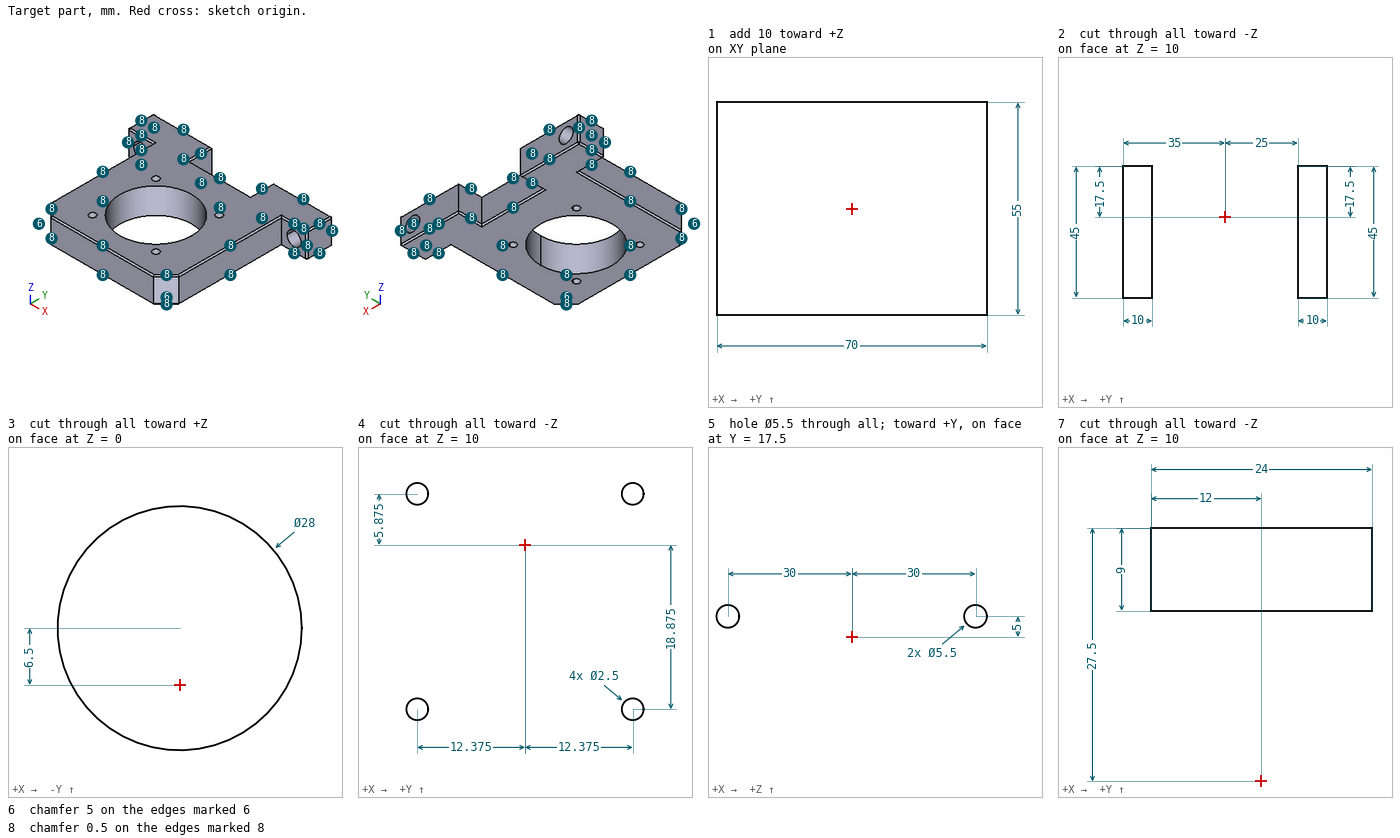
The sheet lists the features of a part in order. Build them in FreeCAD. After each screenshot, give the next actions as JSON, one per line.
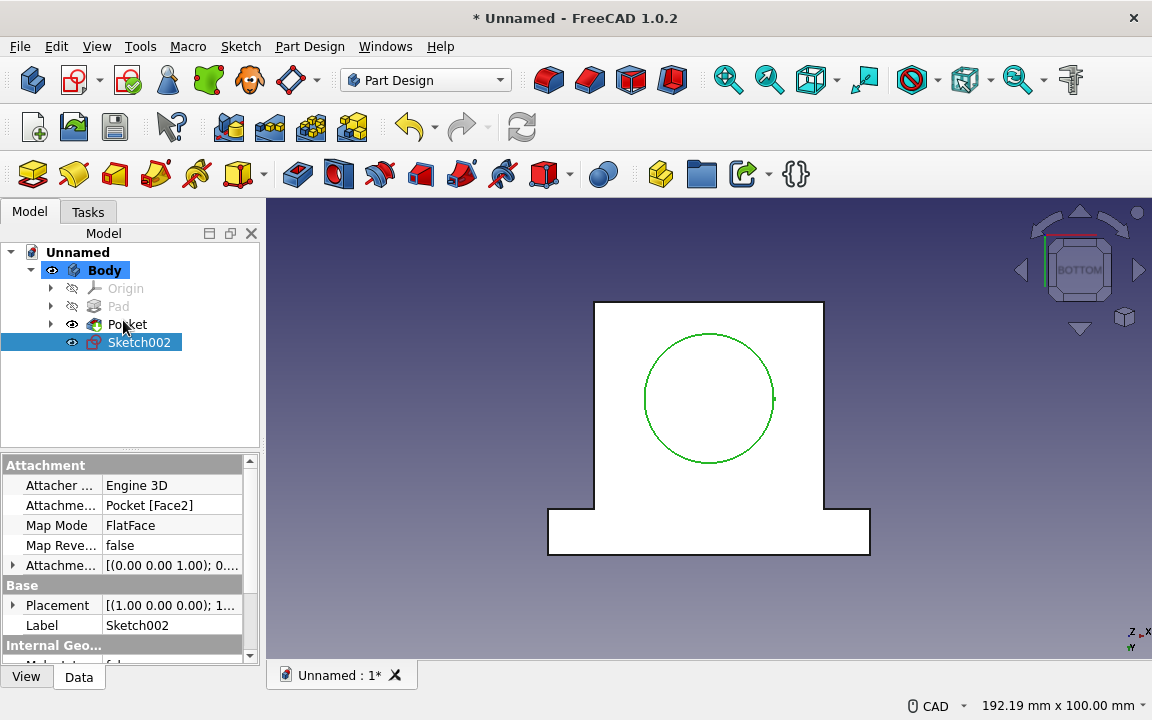
{"action": "left_click", "coordinate": [298, 174]}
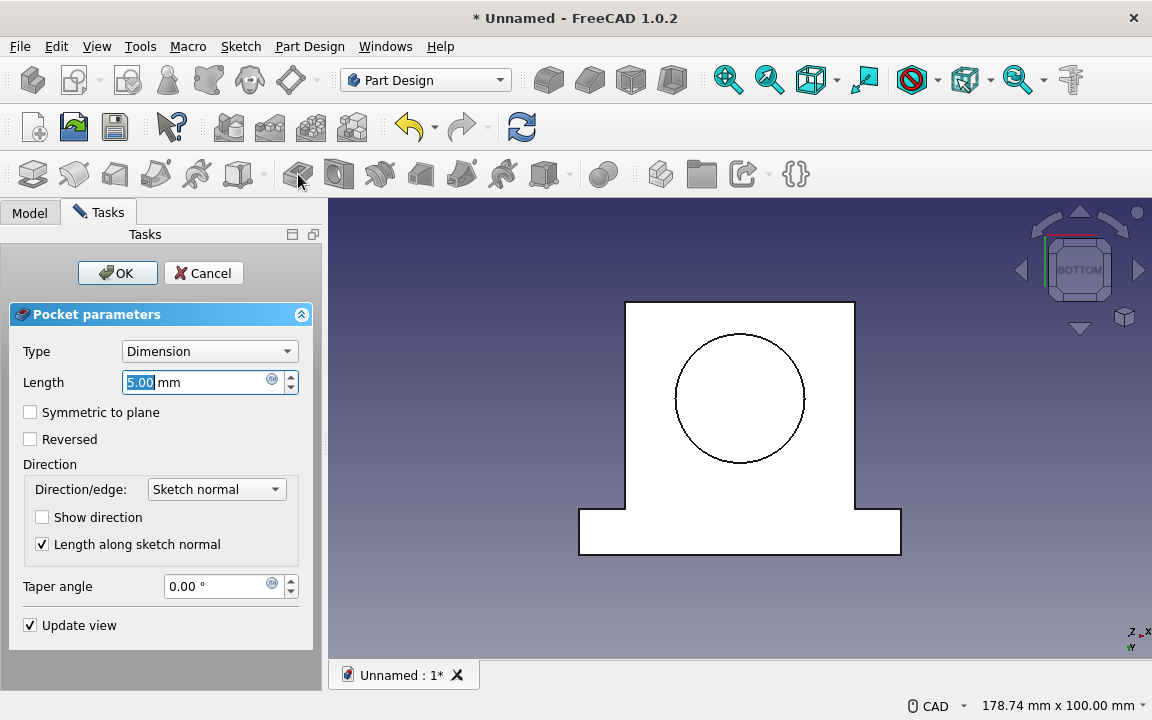
{"action": "left_click", "coordinate": [210, 352]}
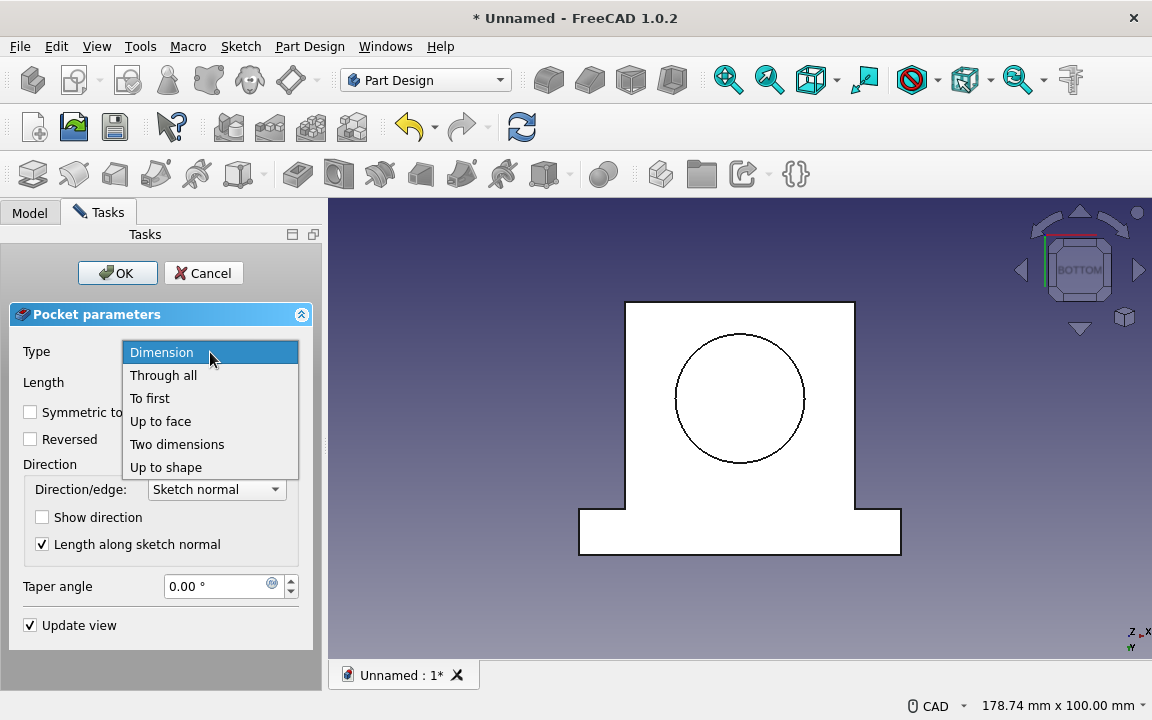
{"action": "left_click", "coordinate": [208, 376]}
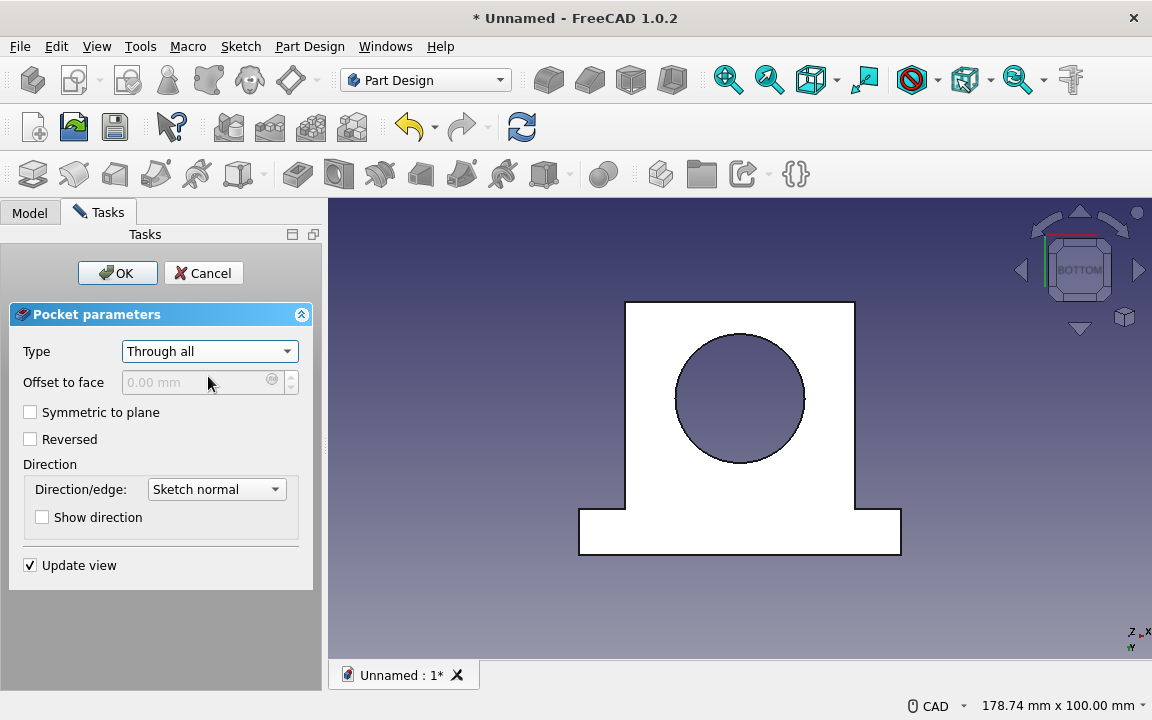
{"action": "left_click", "coordinate": [118, 273]}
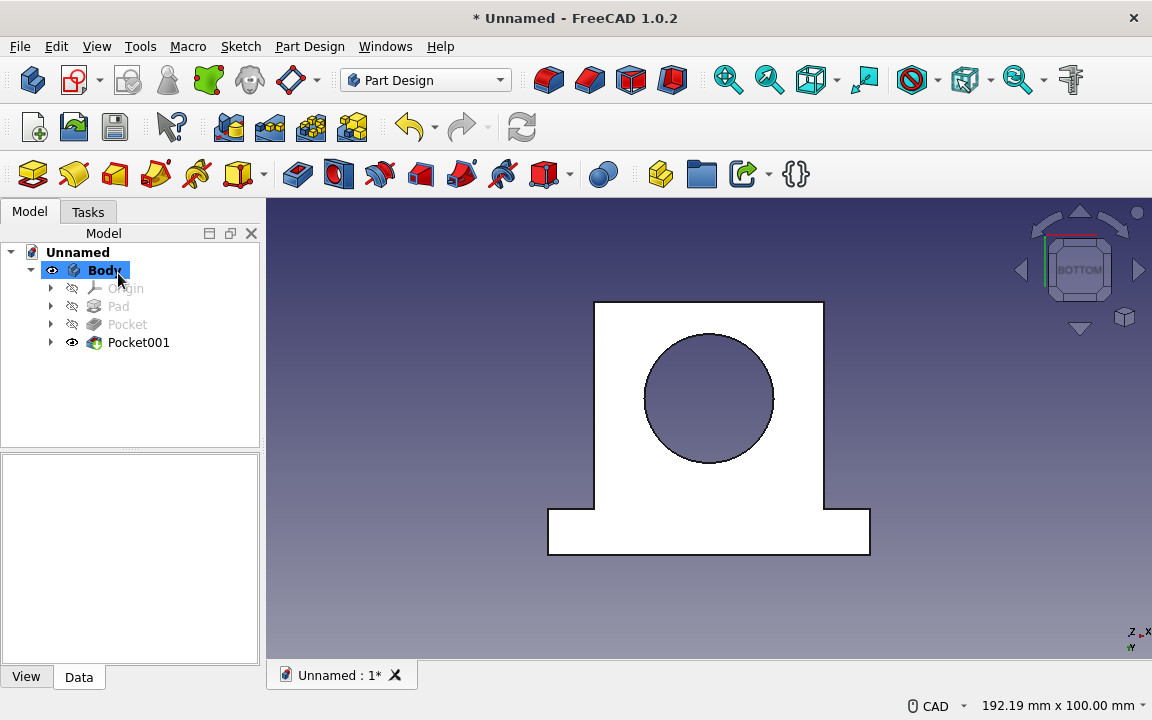
{"action": "key", "text": "0"}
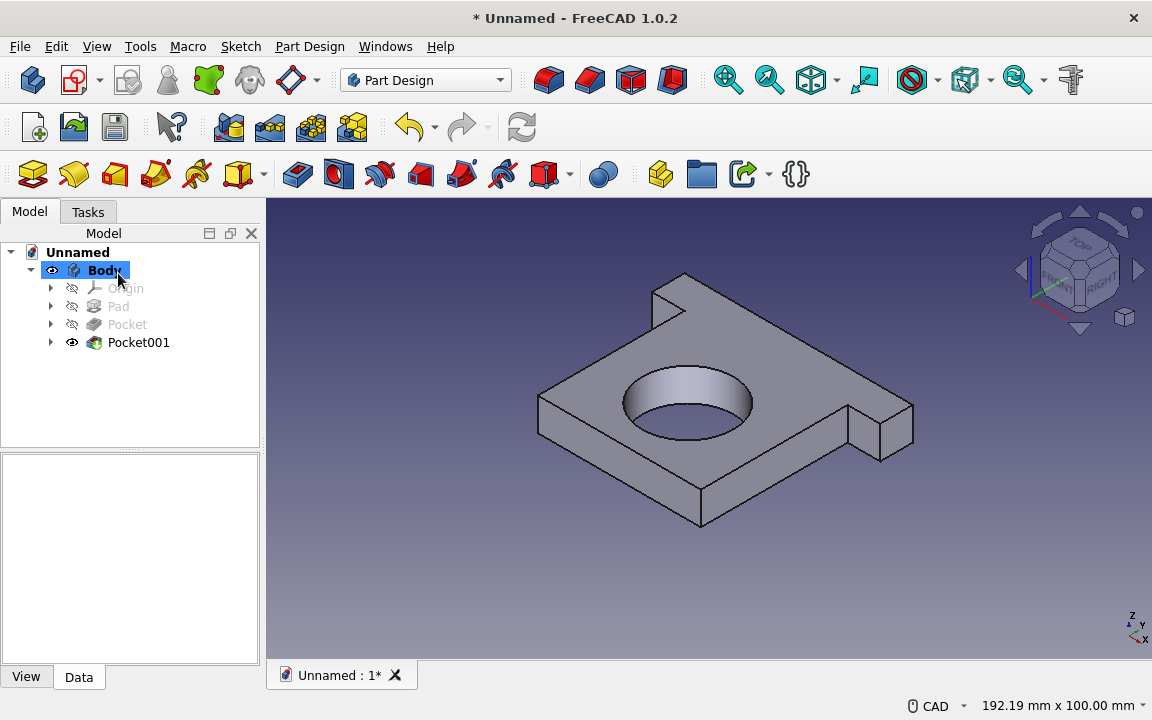
{"action": "left_click", "coordinate": [728, 341]}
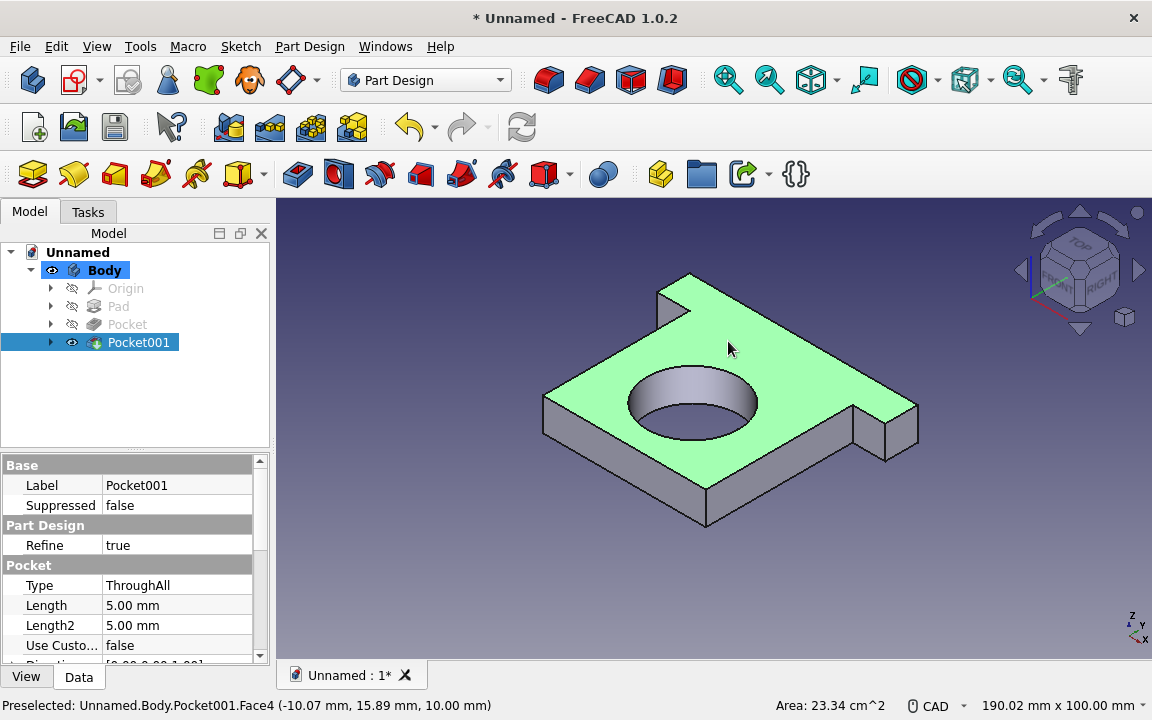
{"action": "left_click", "coordinate": [74, 80]}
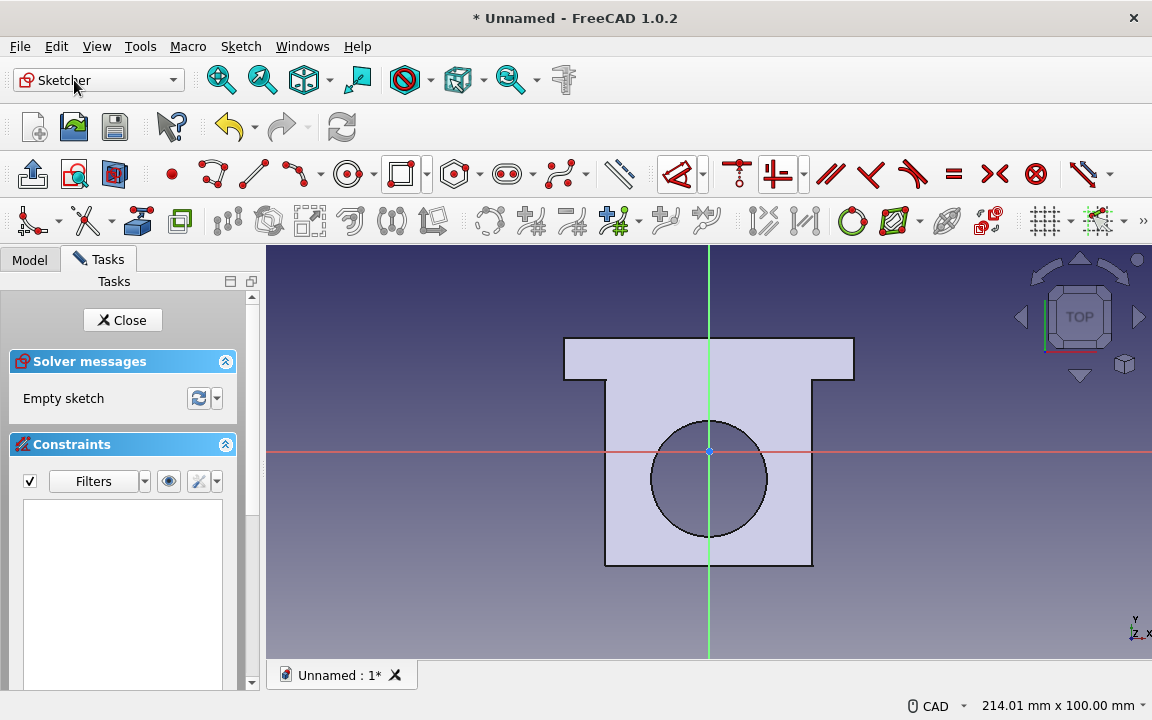
{"action": "scroll", "coordinate": [765, 501], "scroll_direction": "up", "scroll_amount": 4}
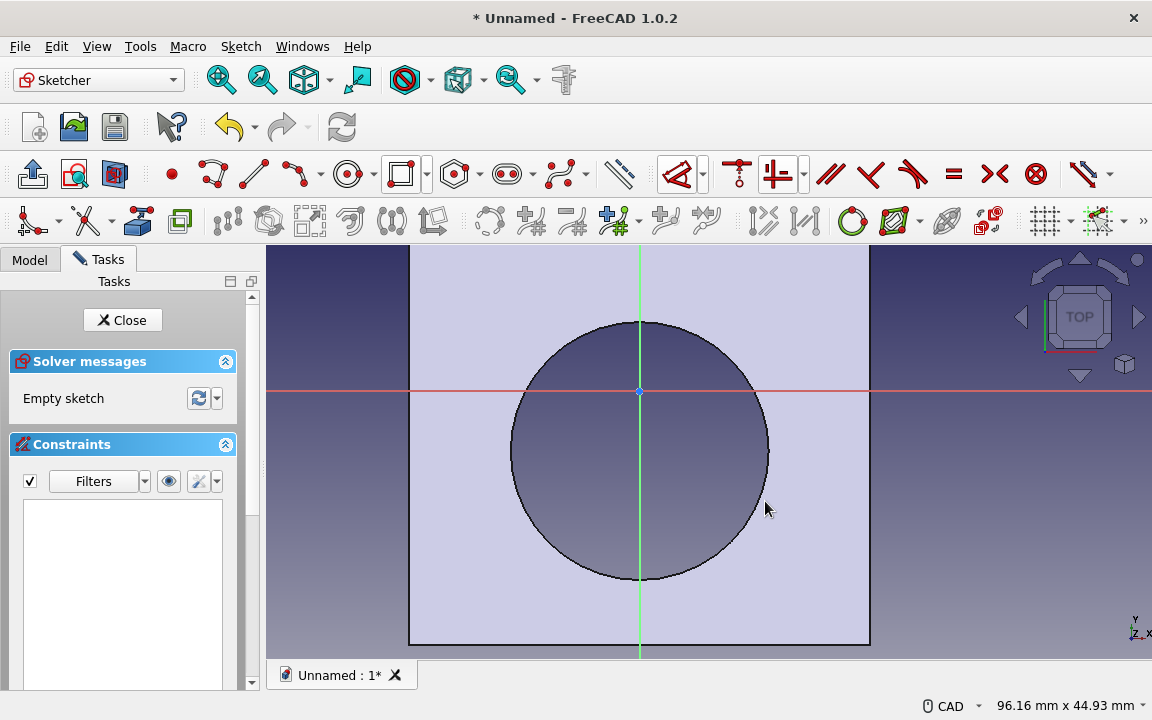
{"action": "left_click", "coordinate": [348, 174]}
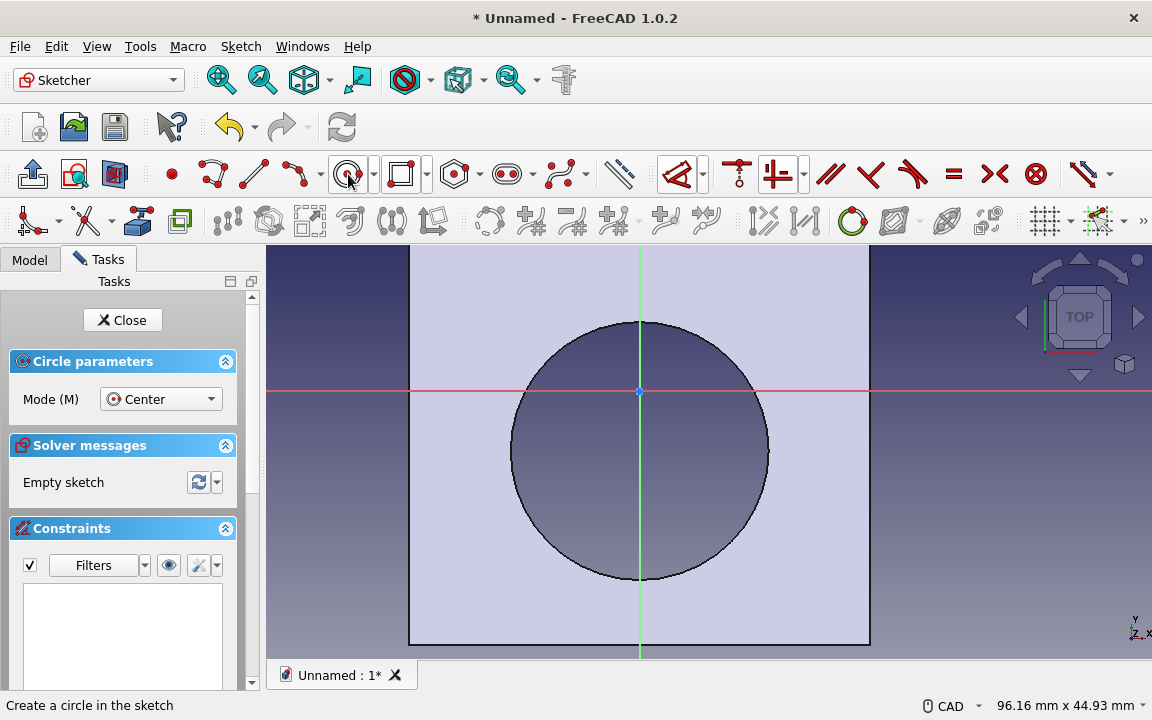
{"action": "scroll", "coordinate": [754, 565], "scroll_direction": "up", "scroll_amount": 4}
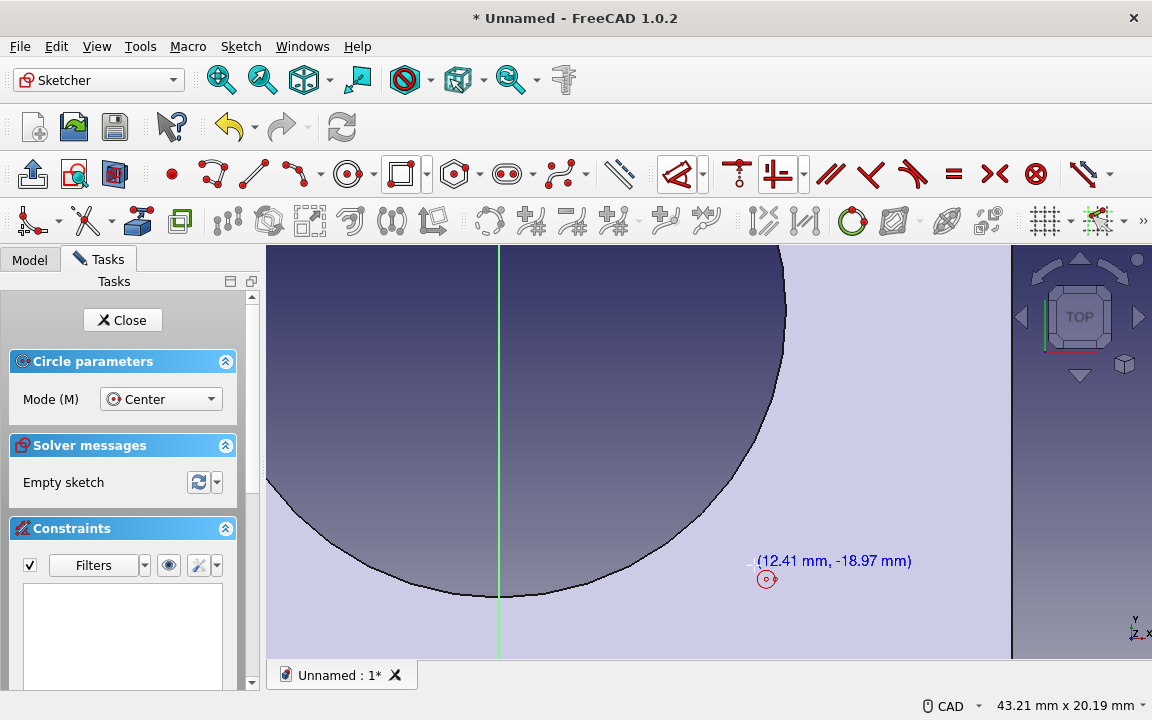
{"action": "left_click", "coordinate": [753, 564]}
{"action": "left_click", "coordinate": [771, 546]}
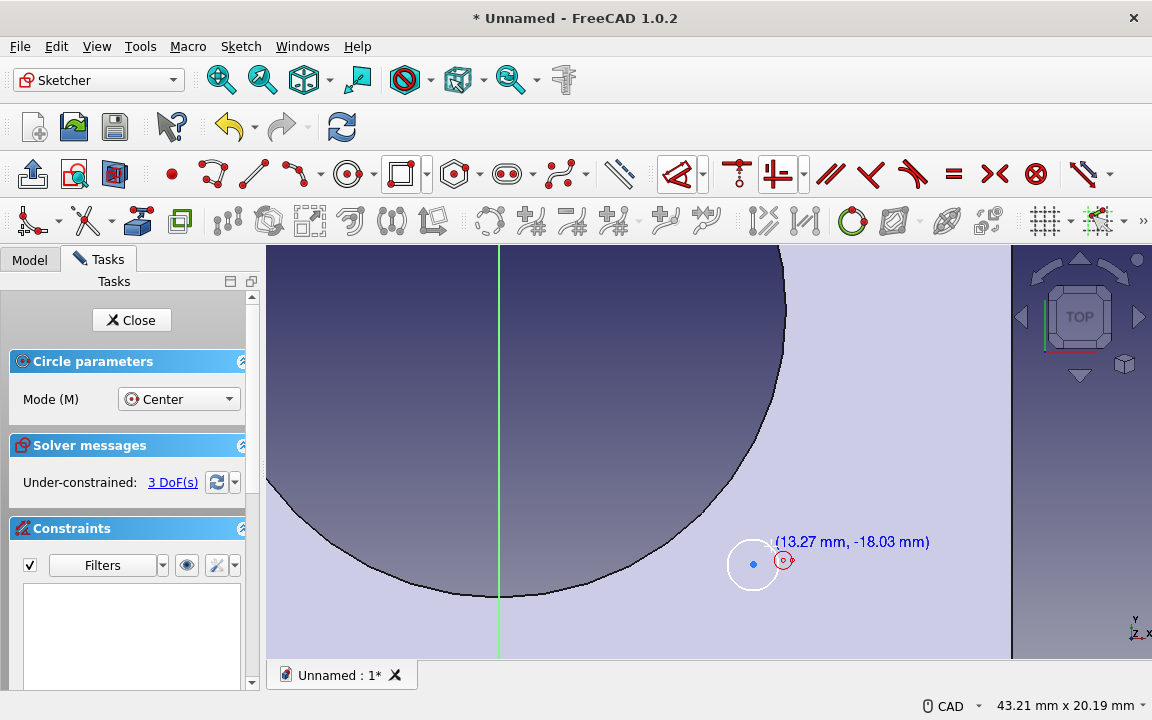
{"action": "scroll", "coordinate": [756, 567], "scroll_direction": "down", "scroll_amount": 4}